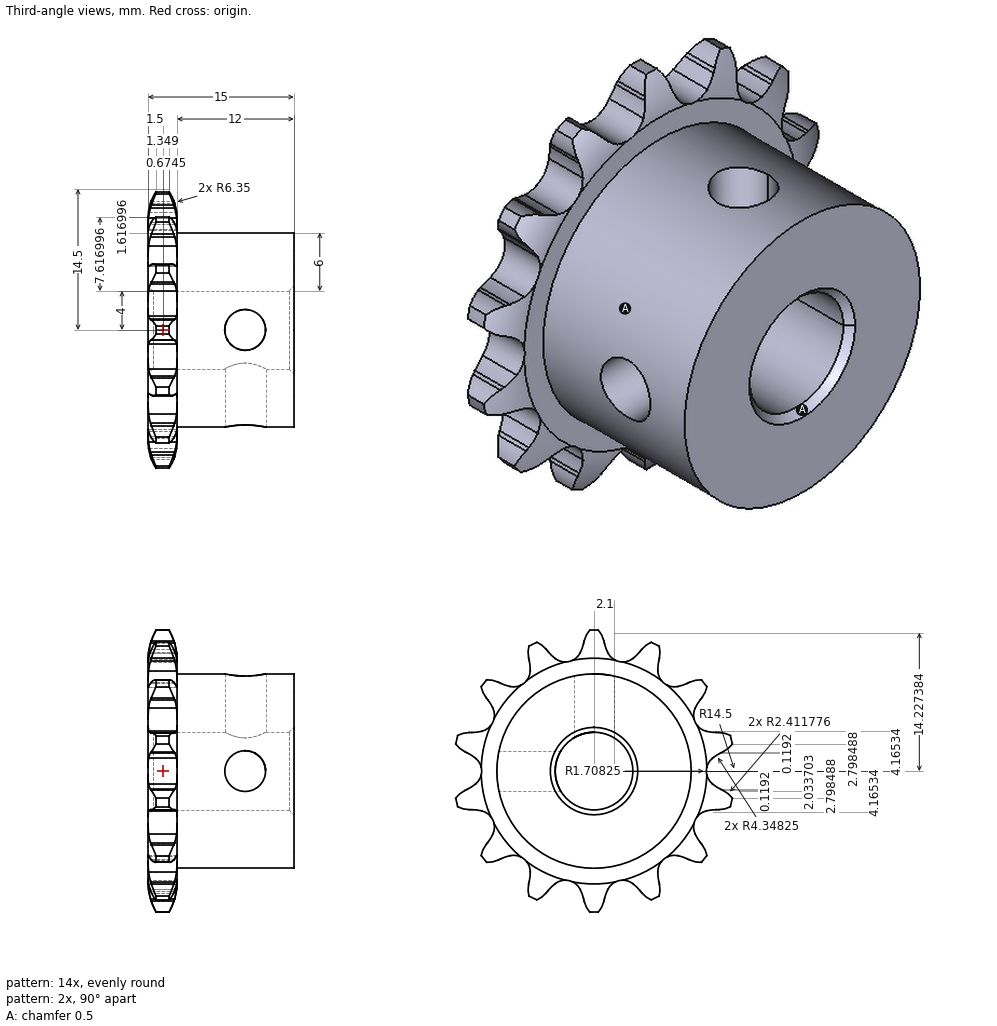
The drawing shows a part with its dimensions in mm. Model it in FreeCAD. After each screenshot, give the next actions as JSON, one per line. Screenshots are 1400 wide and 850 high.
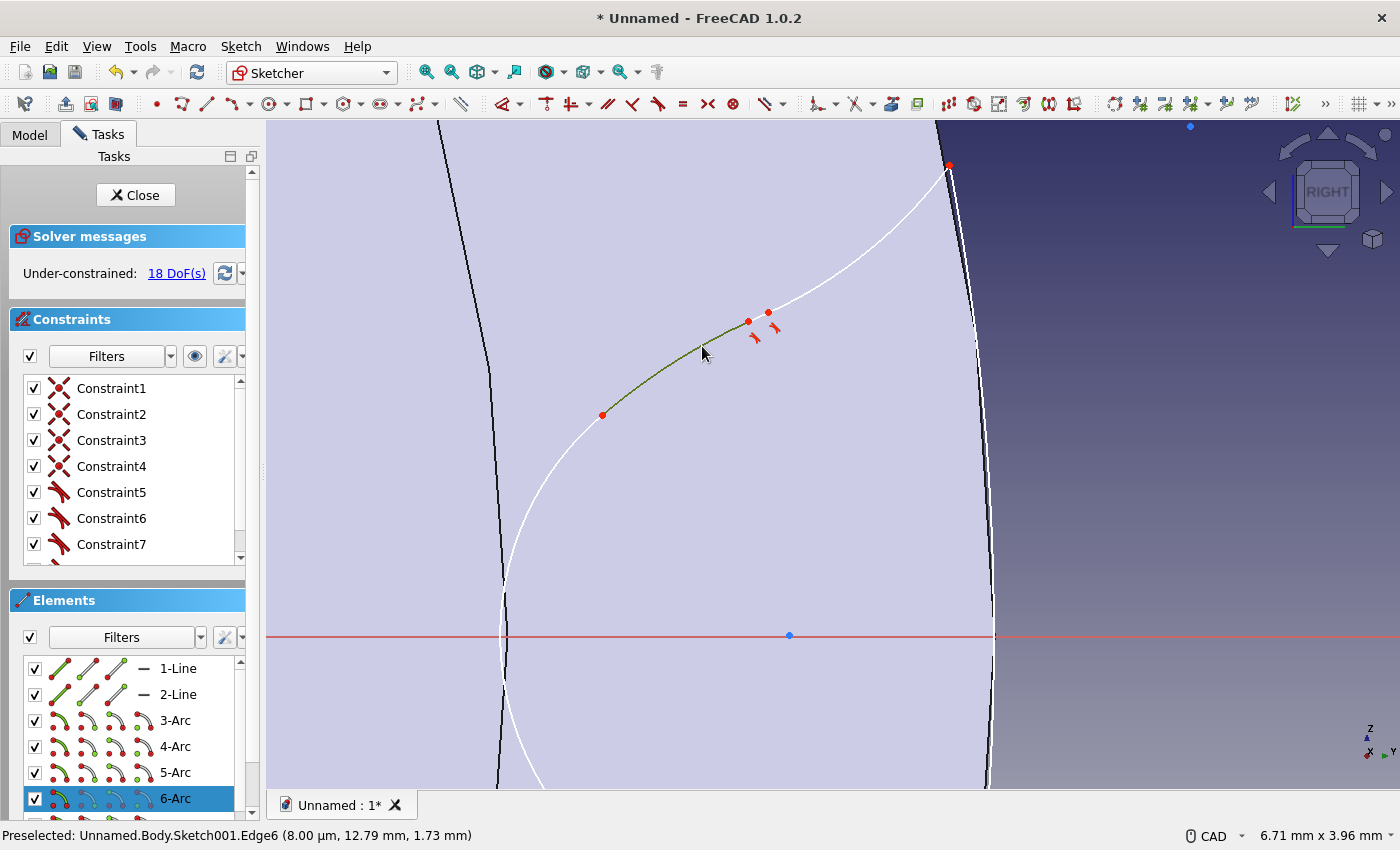
{"action": "left_click", "coordinate": [517, 538]}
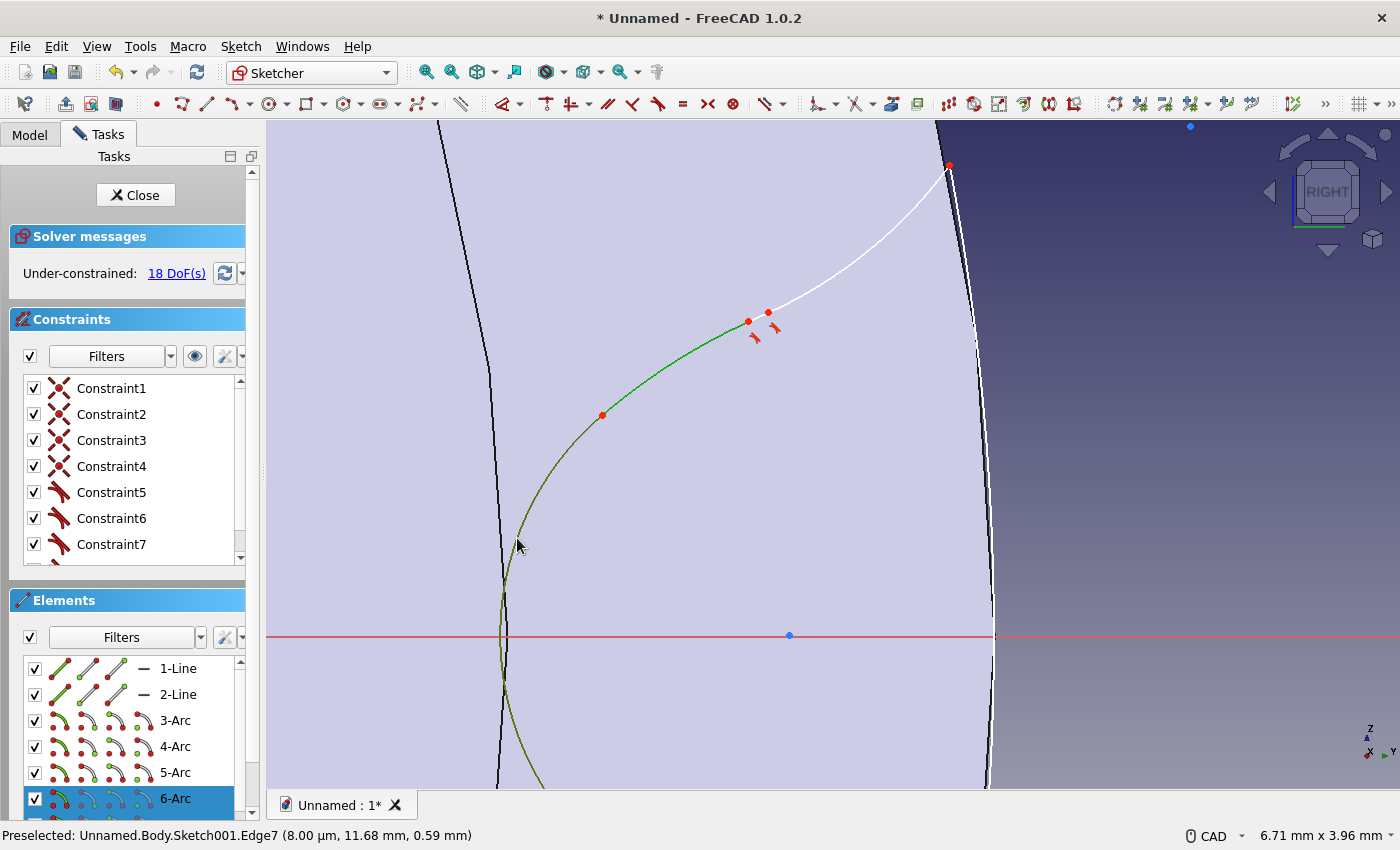
{"action": "left_click", "coordinate": [658, 104]}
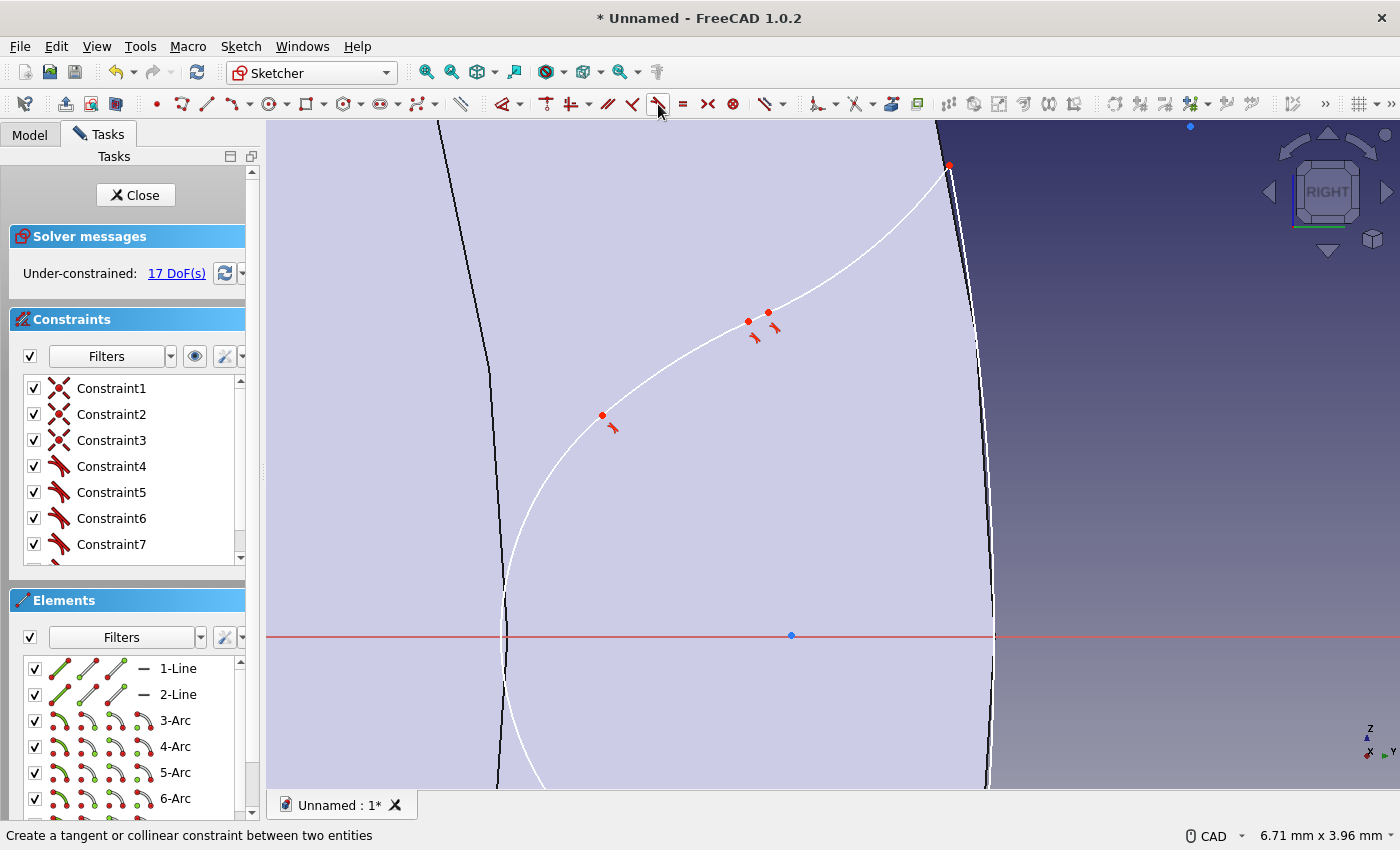
{"action": "left_click", "coordinate": [518, 538]}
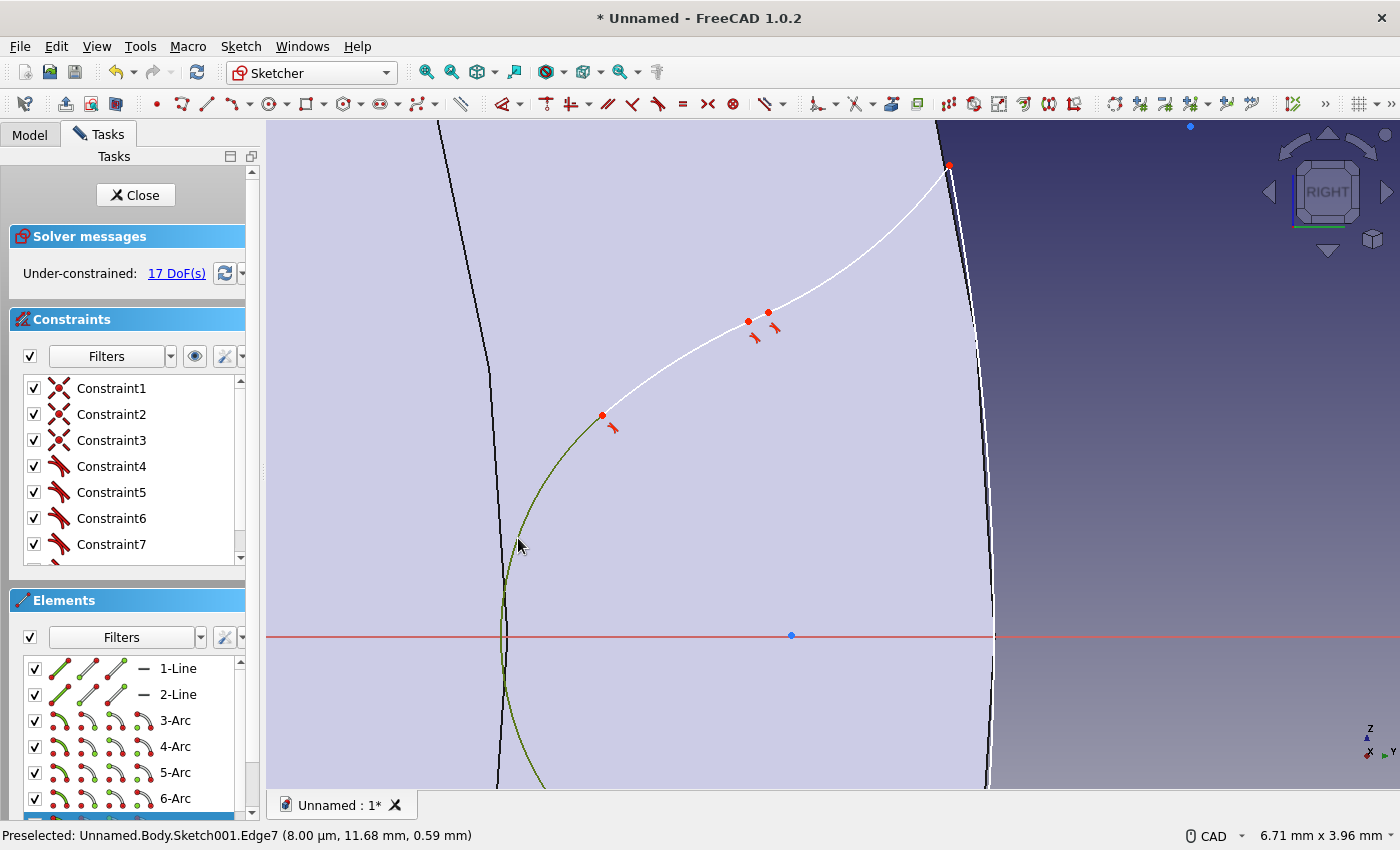
{"action": "scroll", "coordinate": [779, 306], "scroll_direction": "down", "scroll_amount": 4}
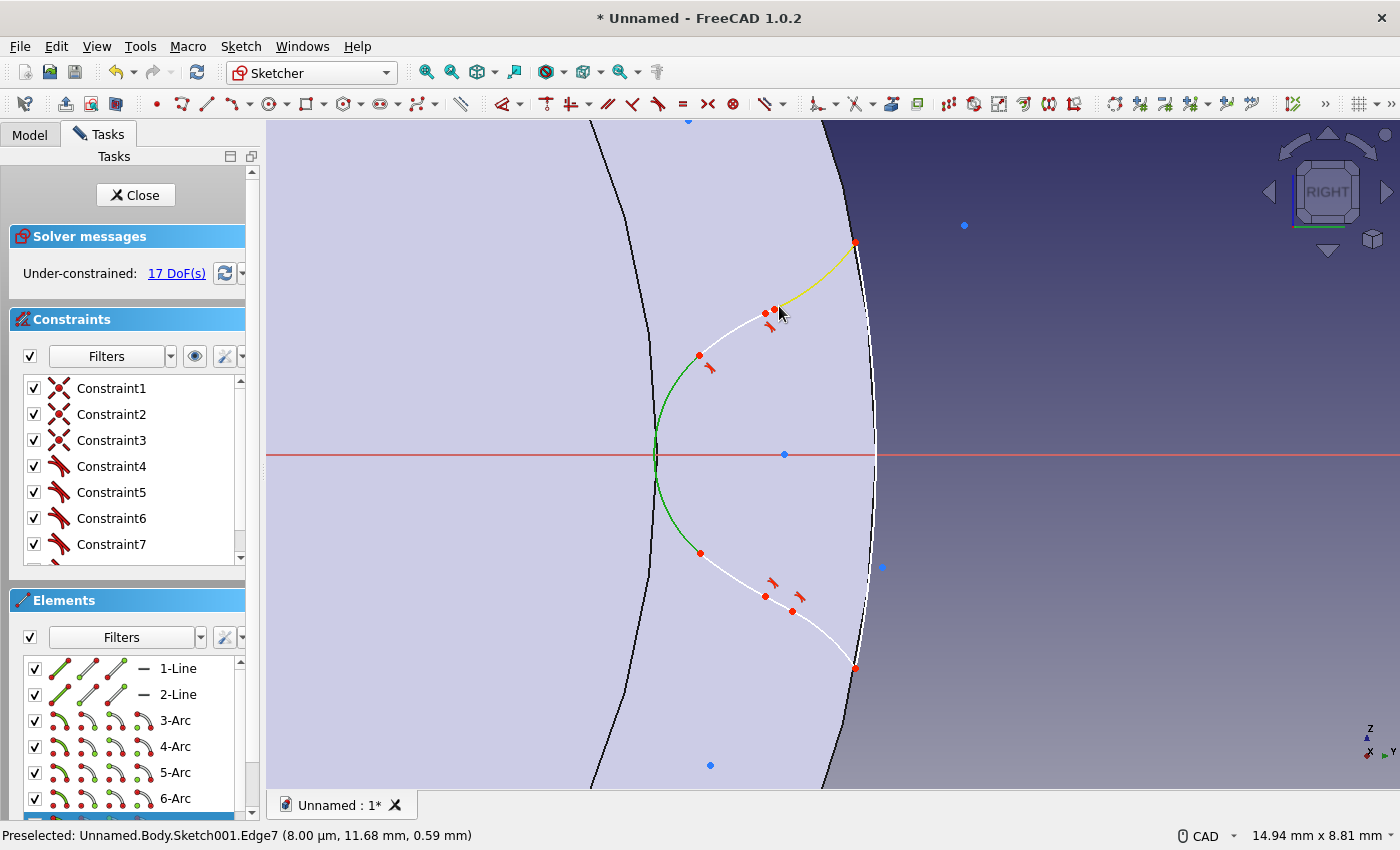
{"action": "left_click", "coordinate": [719, 568]}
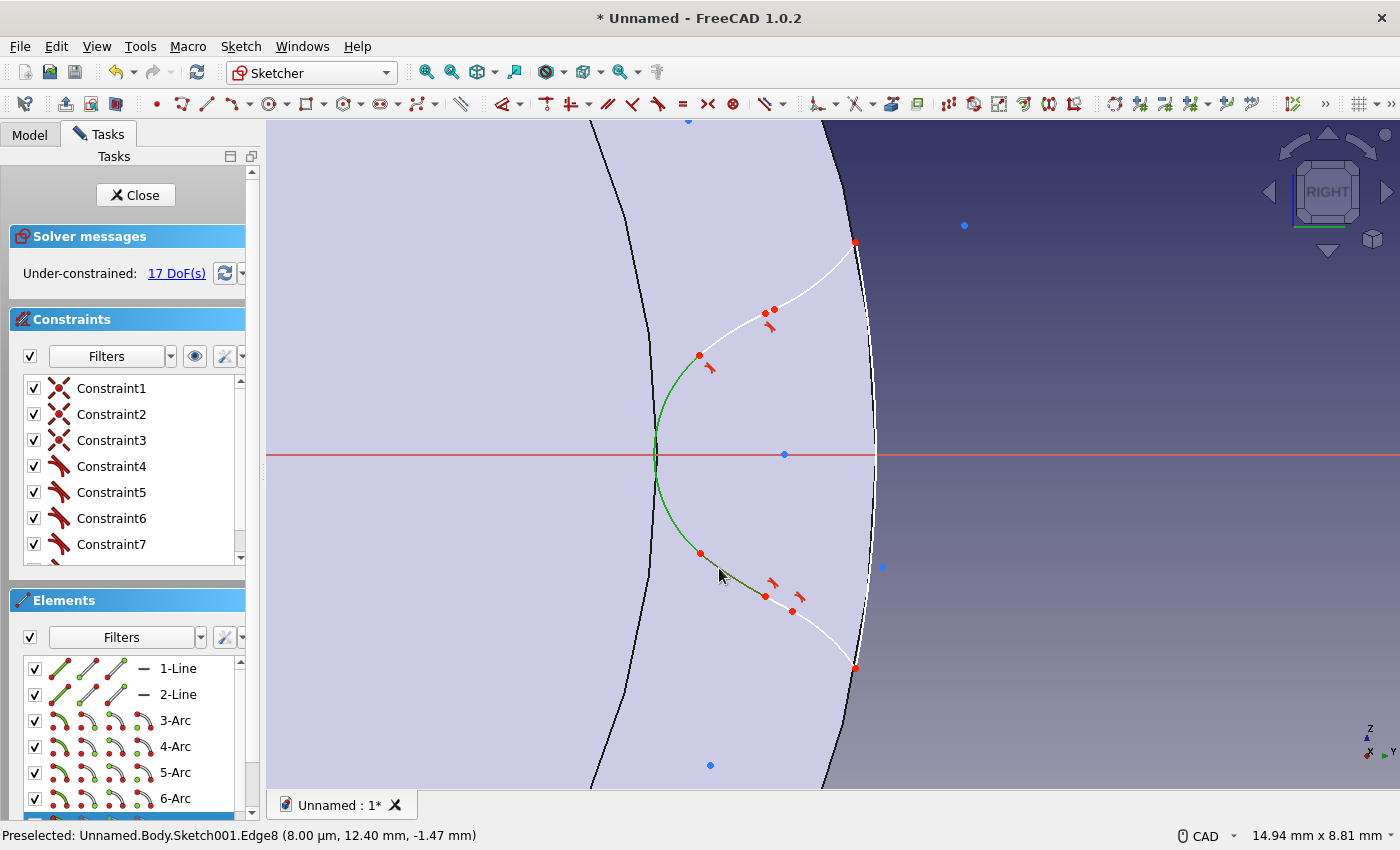
{"action": "left_click", "coordinate": [658, 104]}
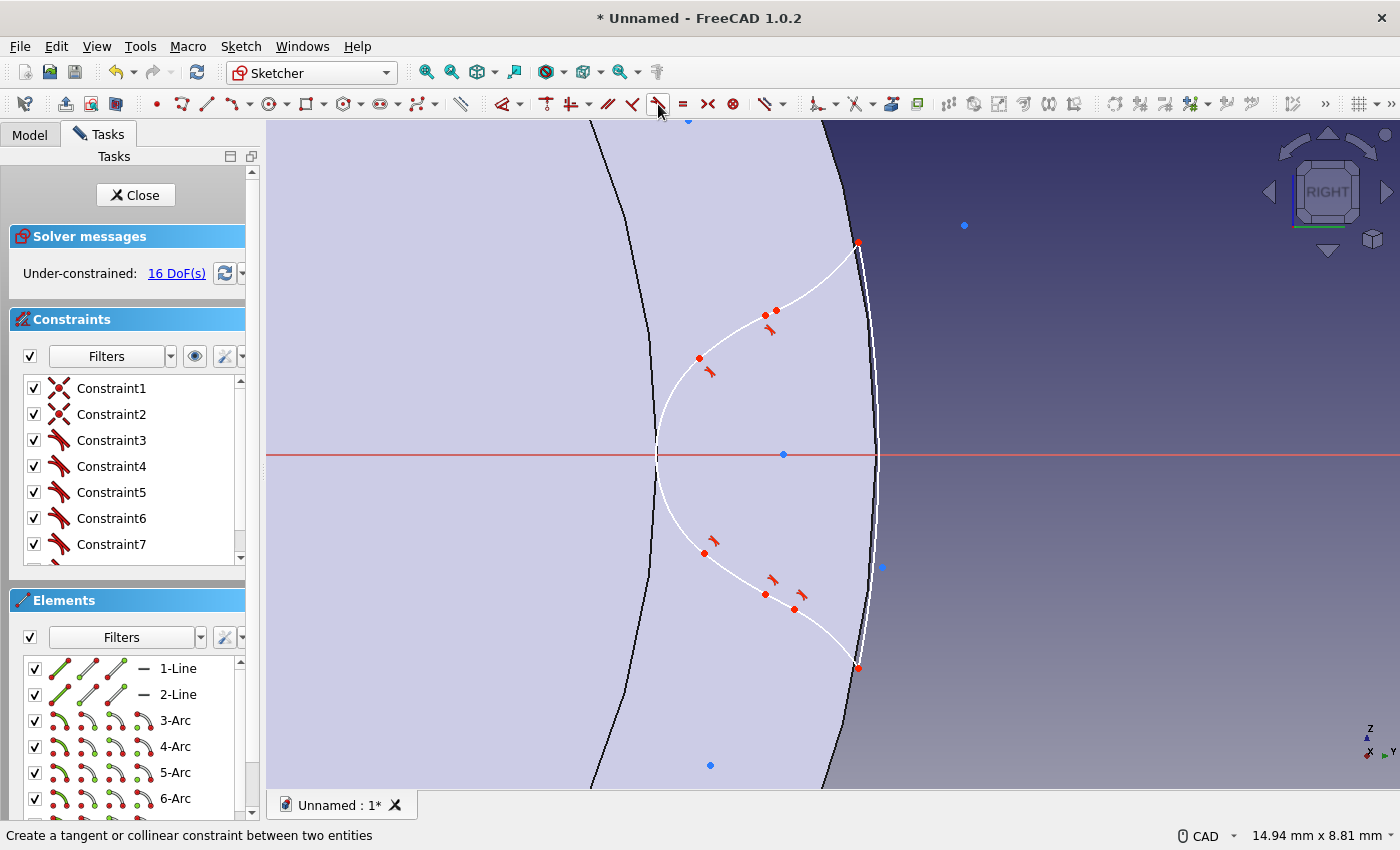
{"action": "scroll", "coordinate": [1235, 454], "scroll_direction": "down", "scroll_amount": 3}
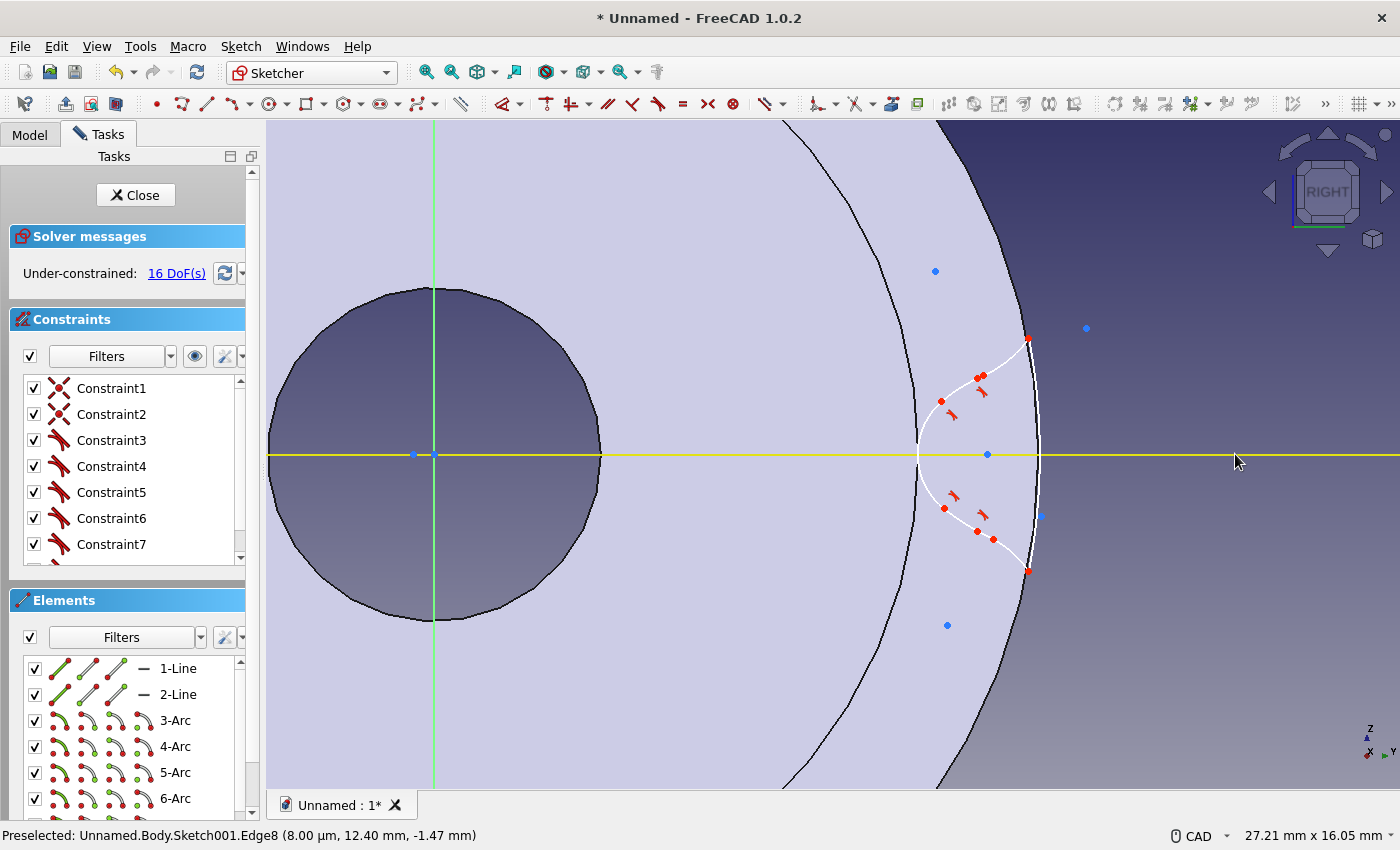
{"action": "left_click_drag", "start_coordinate": [403, 445], "coordinate": [444, 465]}